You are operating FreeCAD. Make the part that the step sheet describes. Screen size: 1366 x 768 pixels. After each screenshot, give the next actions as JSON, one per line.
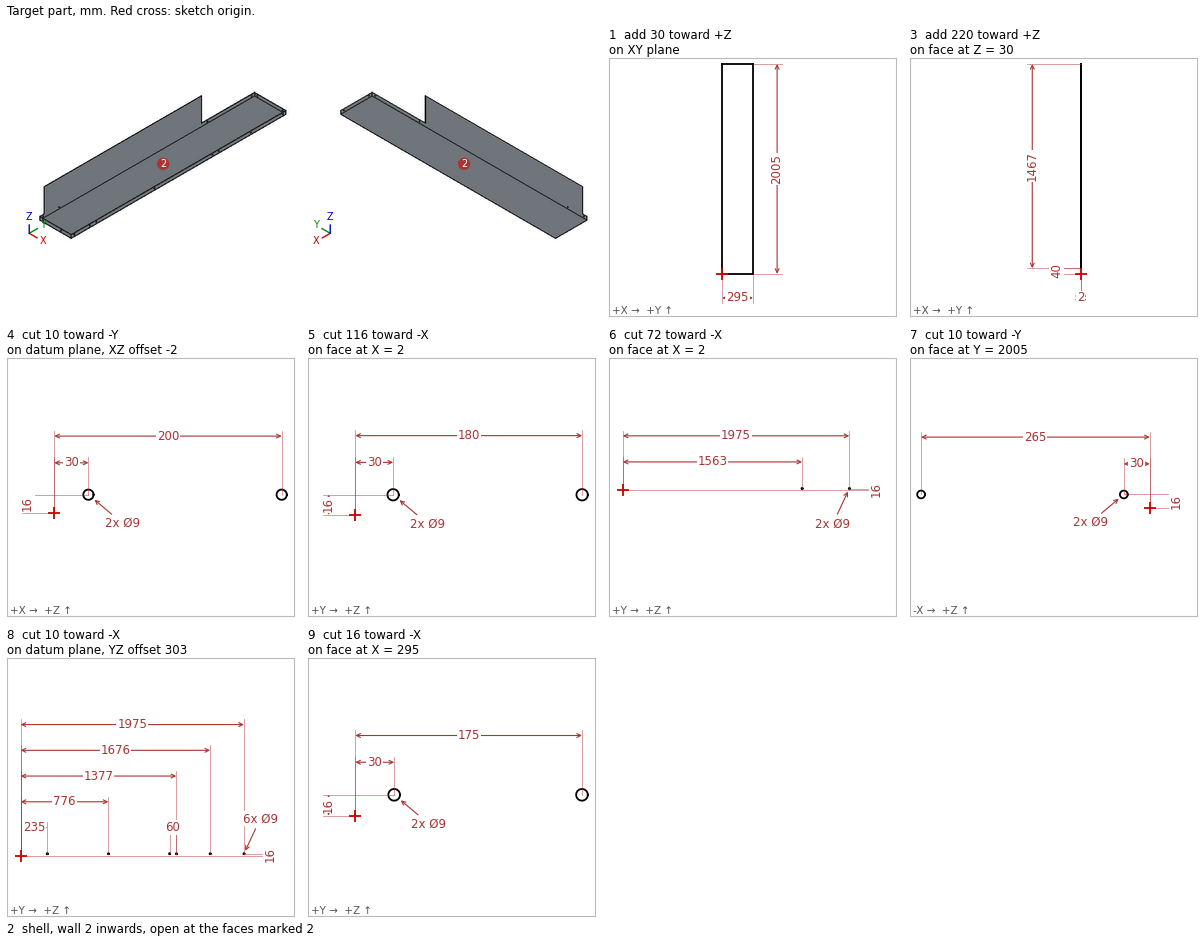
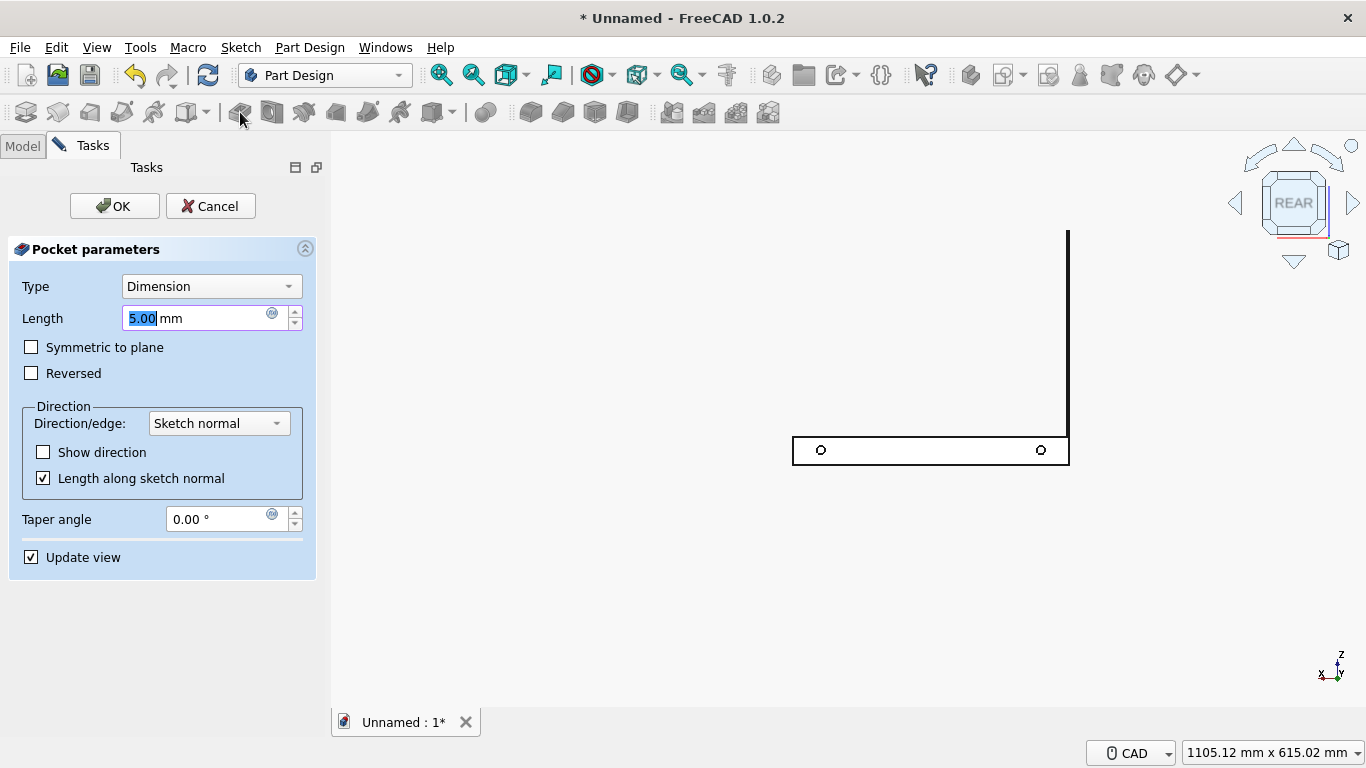
{"action": "type", "text": "10"}
{"action": "key", "text": "Tab"}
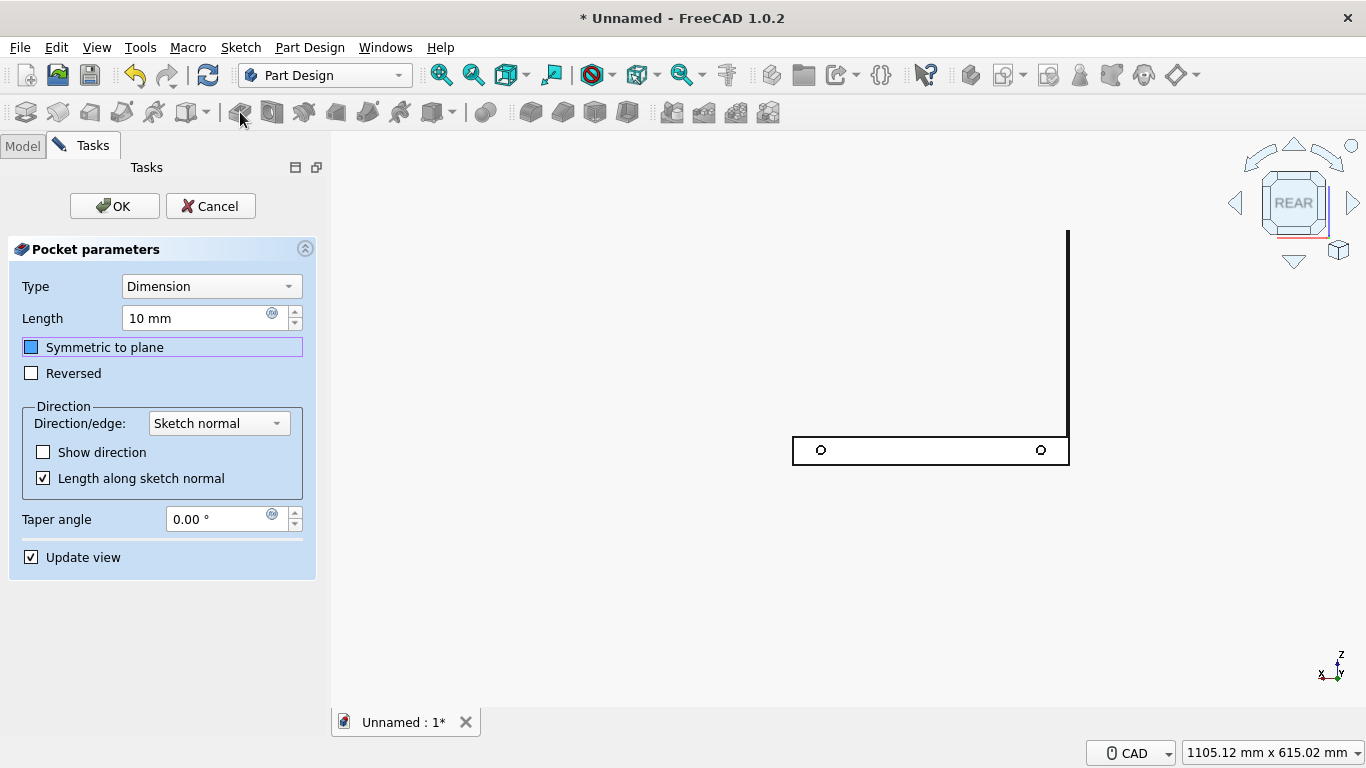
{"action": "left_click", "coordinate": [115, 206]}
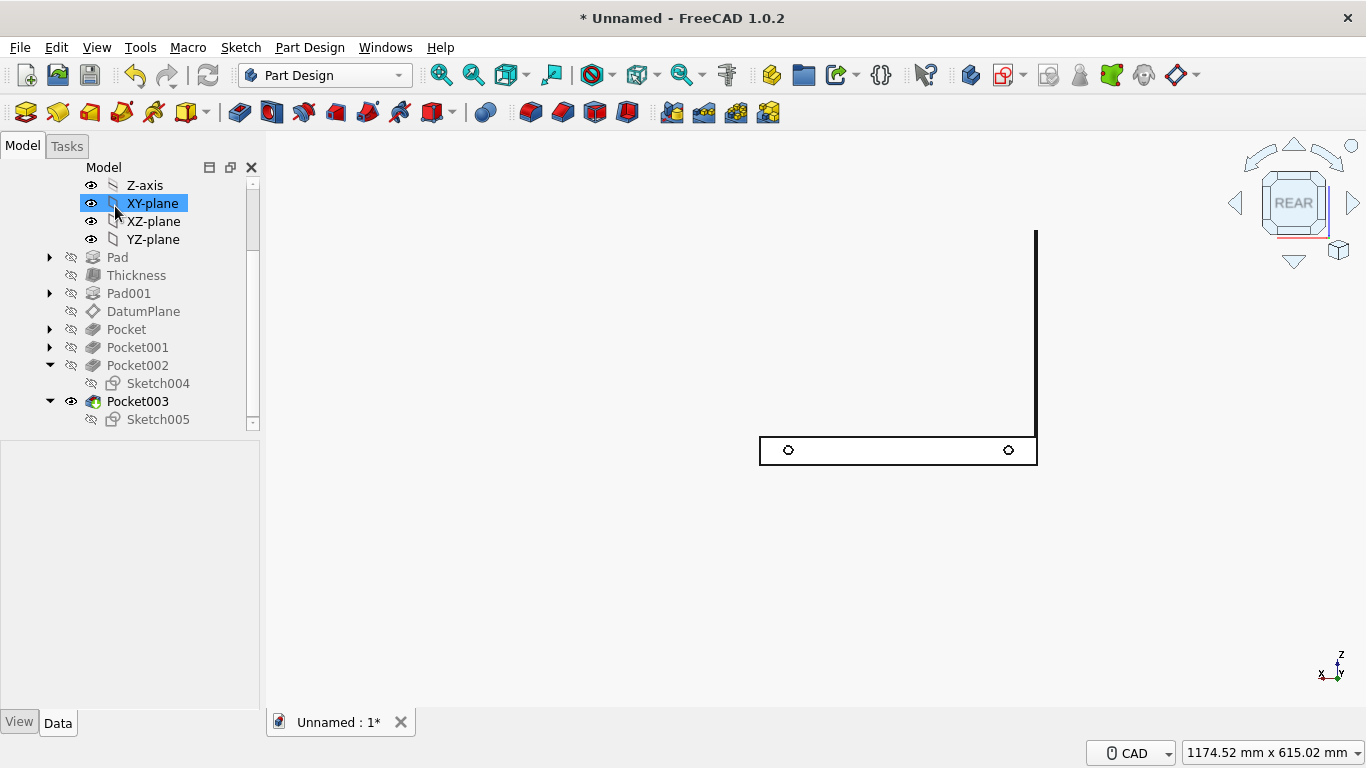
{"action": "key", "text": "v f"}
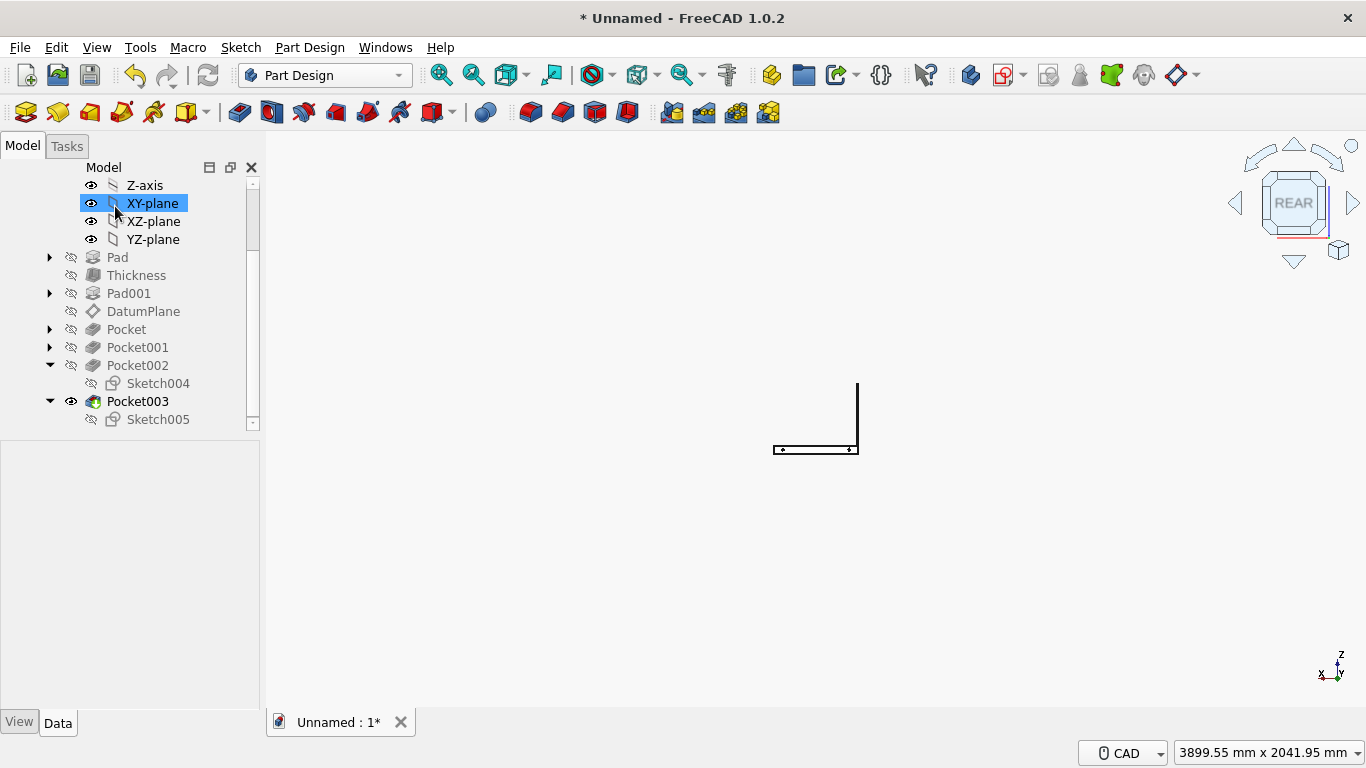
{"action": "scroll", "coordinate": [160, 307], "scroll_direction": "down", "scroll_amount": 3}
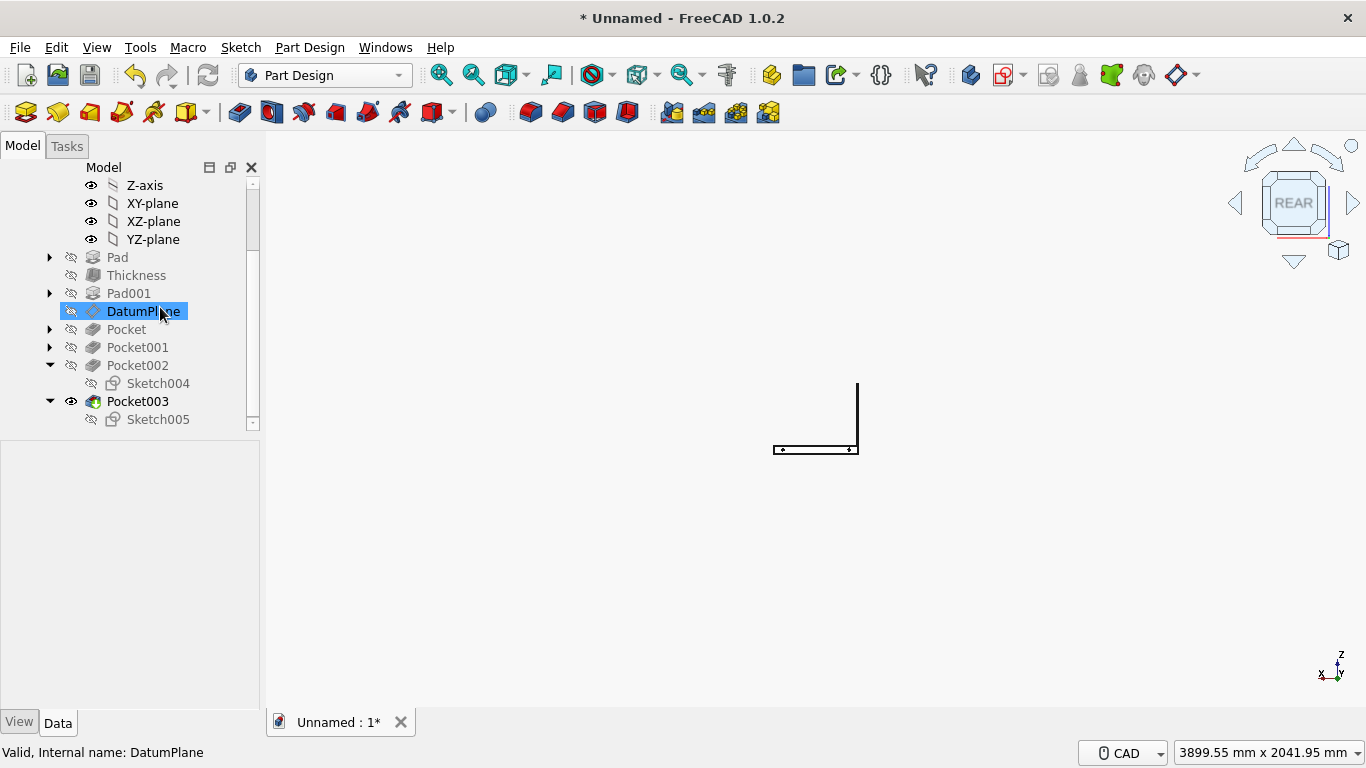
{"action": "scroll", "coordinate": [160, 307], "scroll_direction": "up", "scroll_amount": 15}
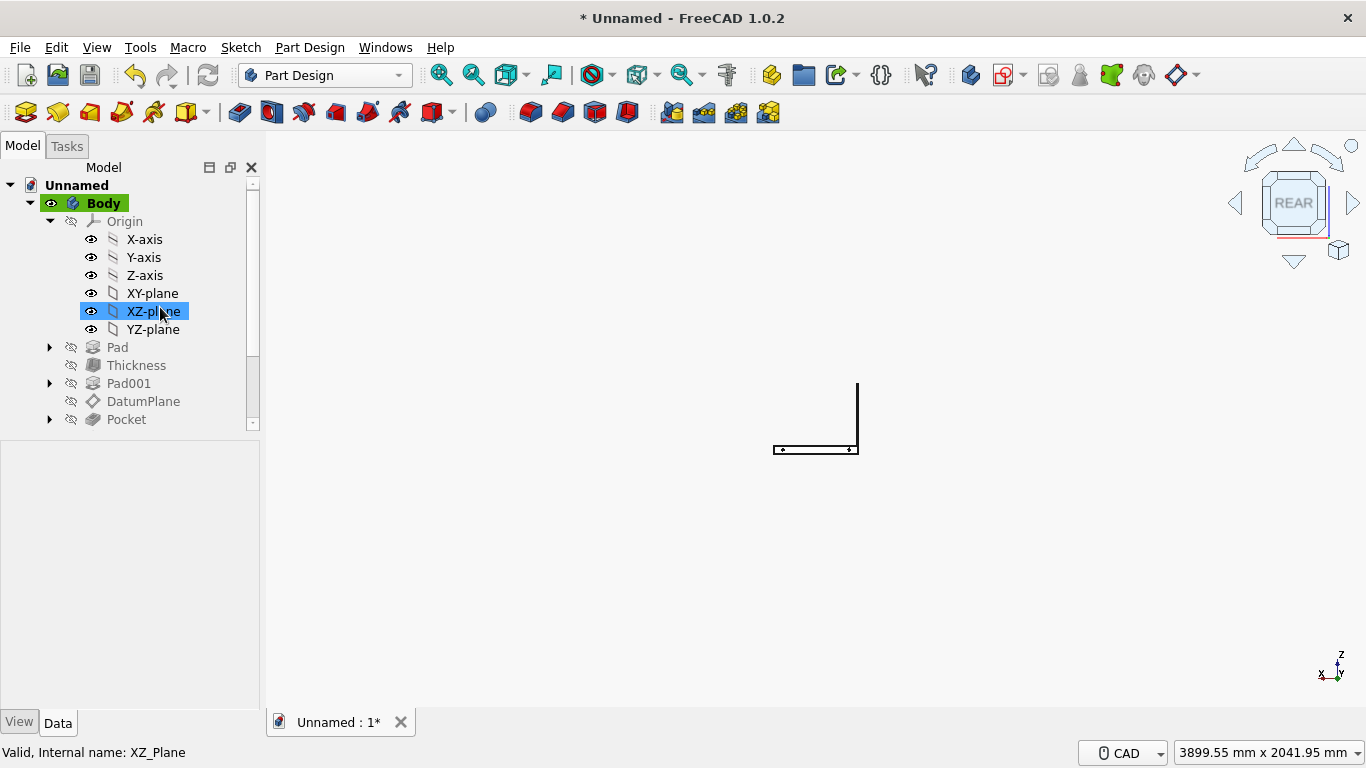
{"action": "left_click", "coordinate": [136, 329]}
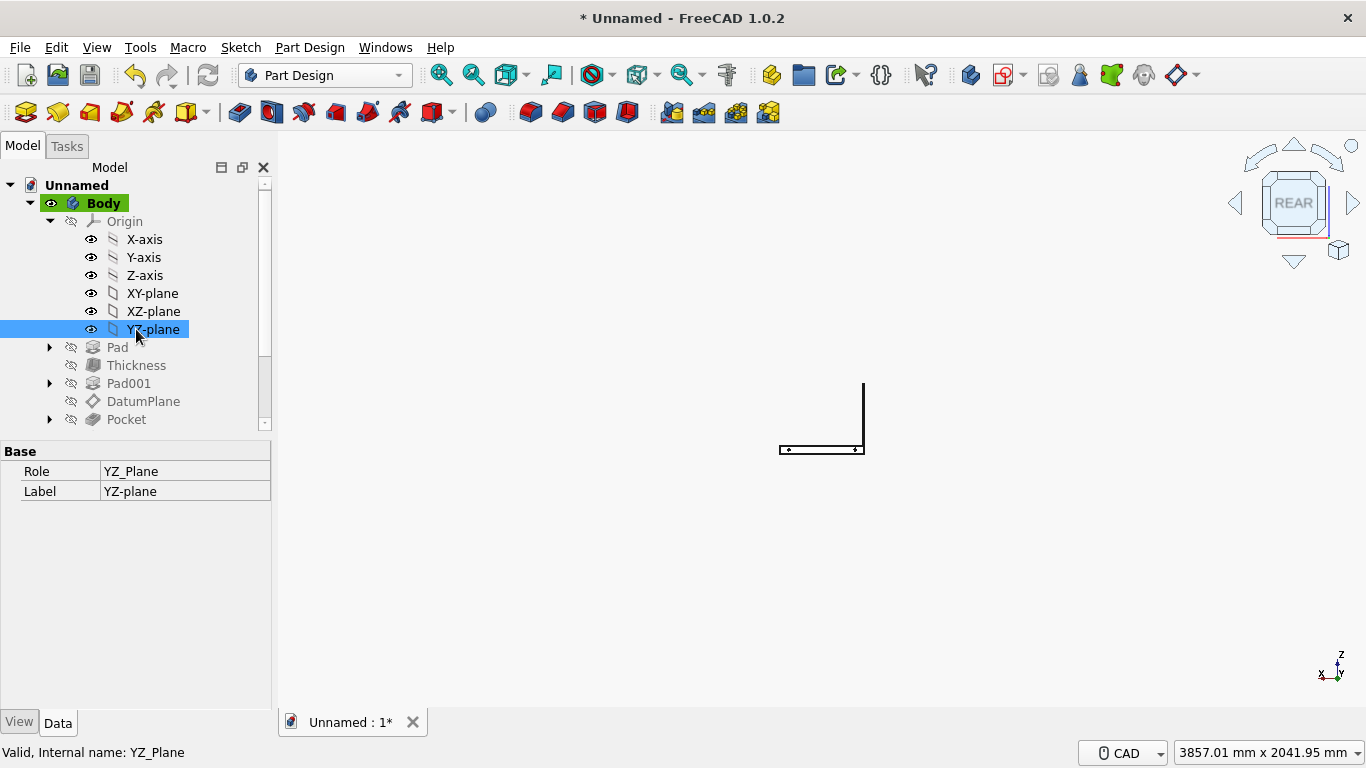
{"action": "left_click", "coordinate": [1176, 76]}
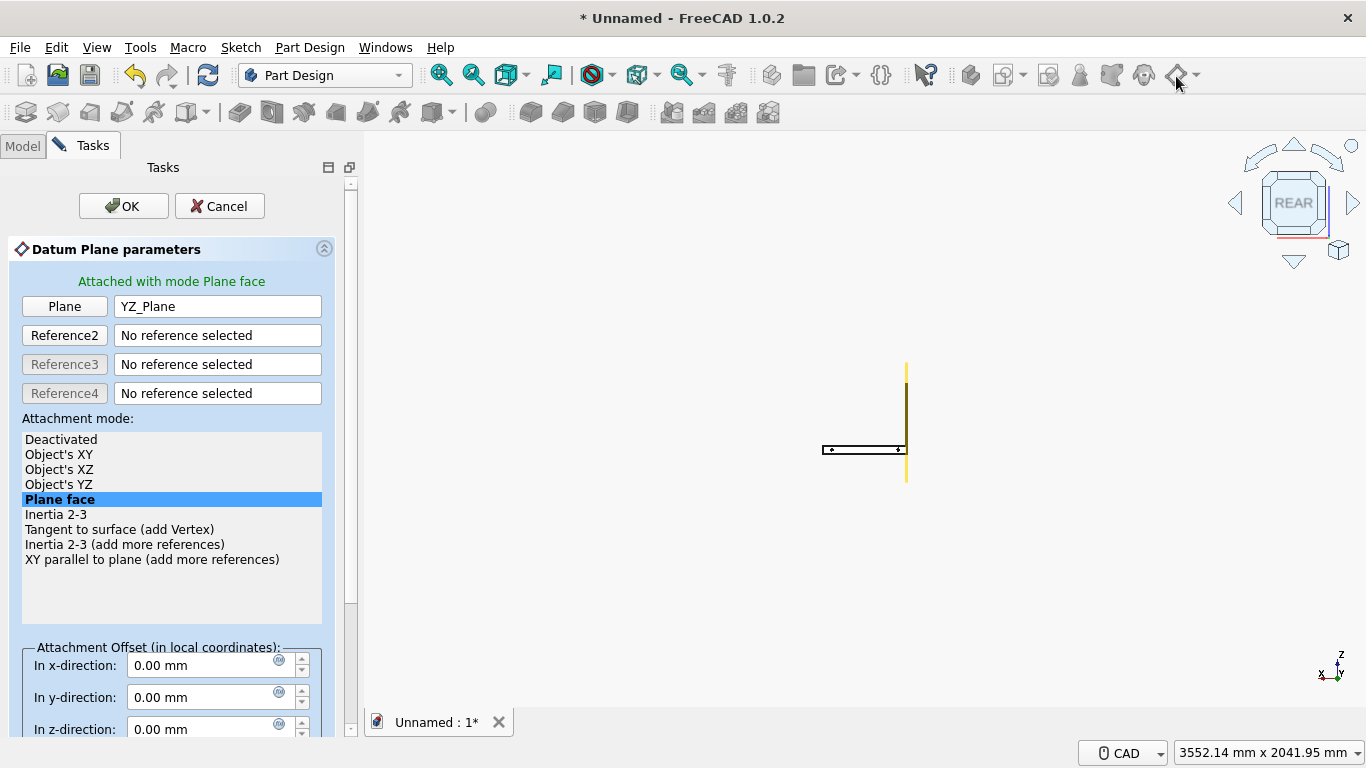
{"action": "scroll", "coordinate": [351, 456], "scroll_direction": "down", "scroll_amount": 2}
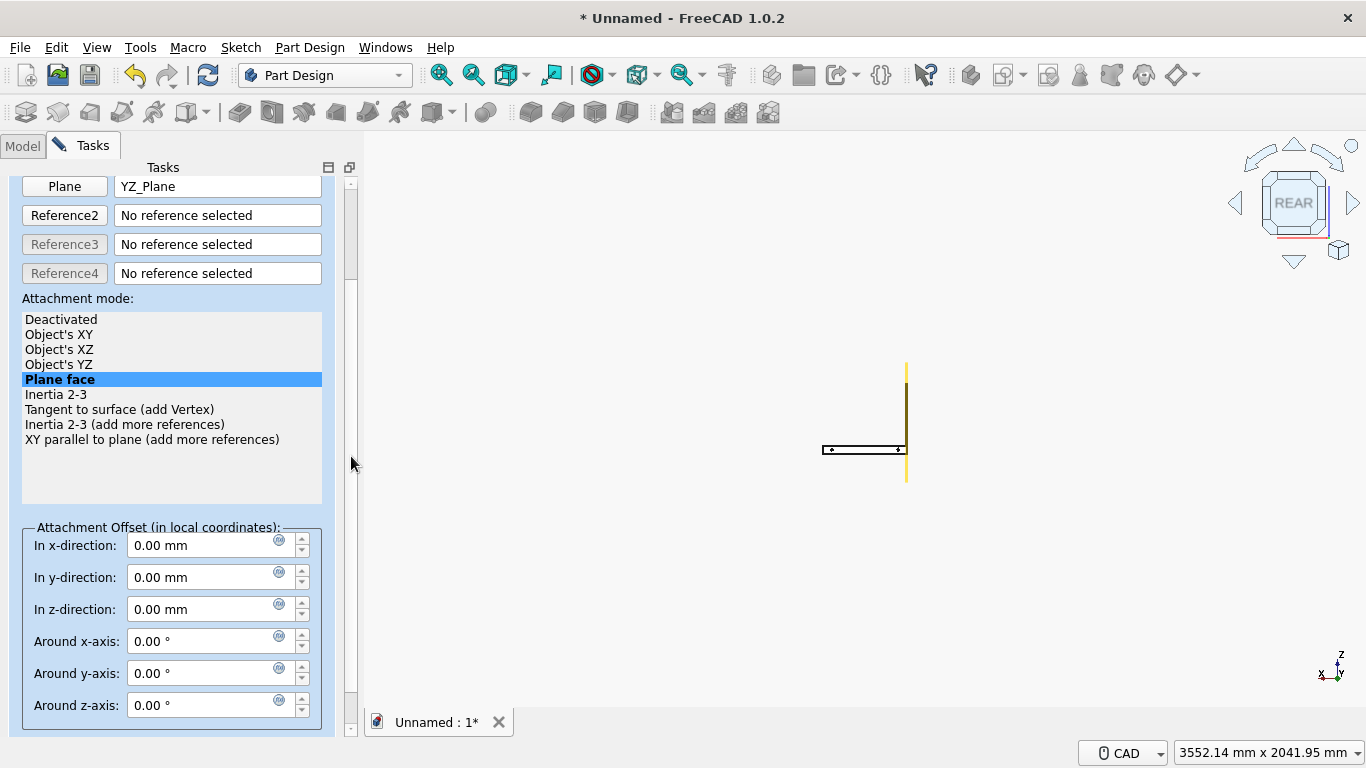
{"action": "triple_click", "coordinate": [210, 609]}